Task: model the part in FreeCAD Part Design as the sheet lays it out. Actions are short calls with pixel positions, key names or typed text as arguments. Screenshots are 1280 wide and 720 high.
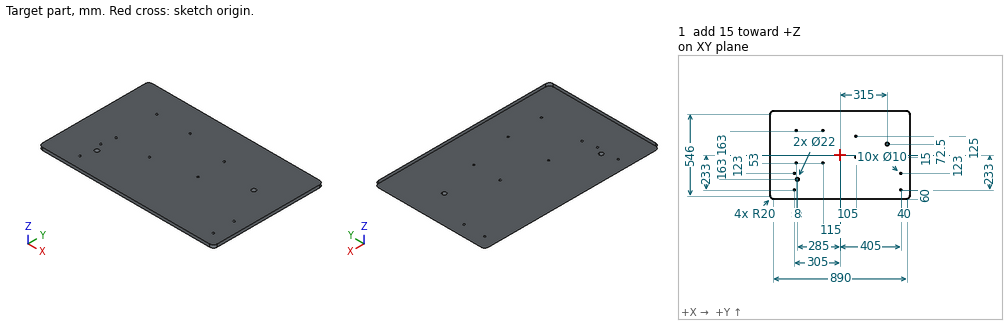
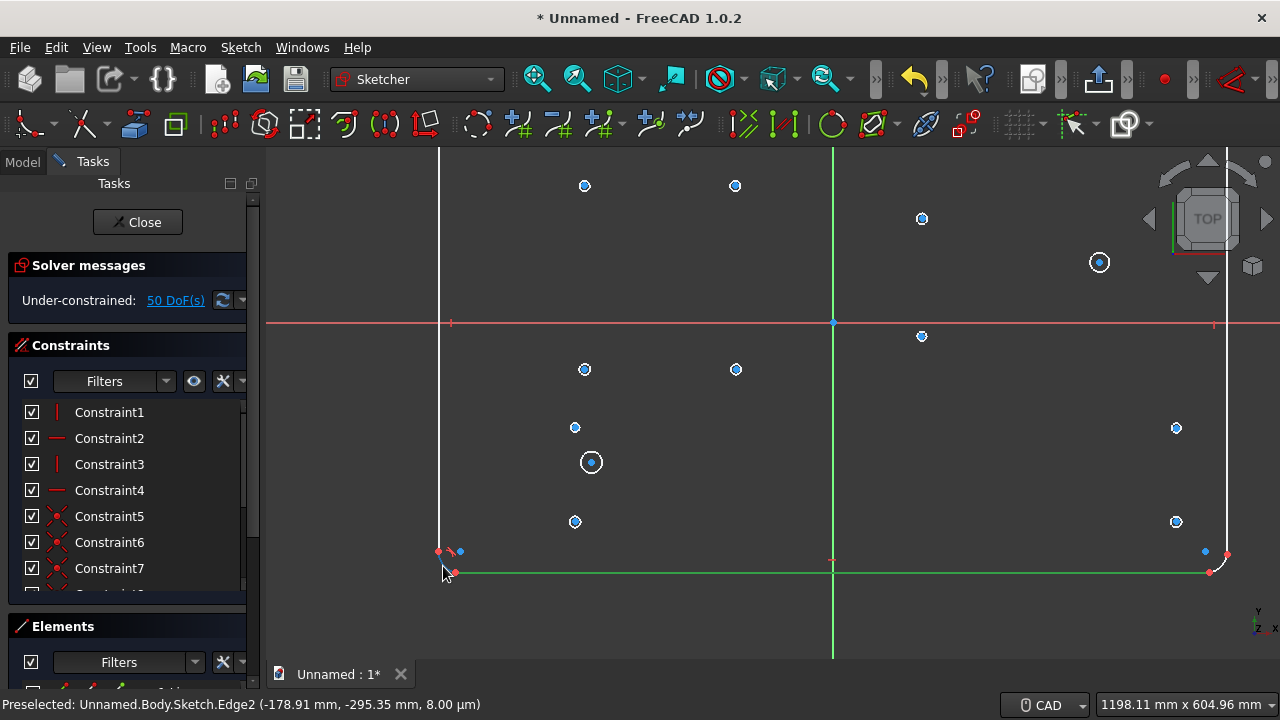
click(443, 565)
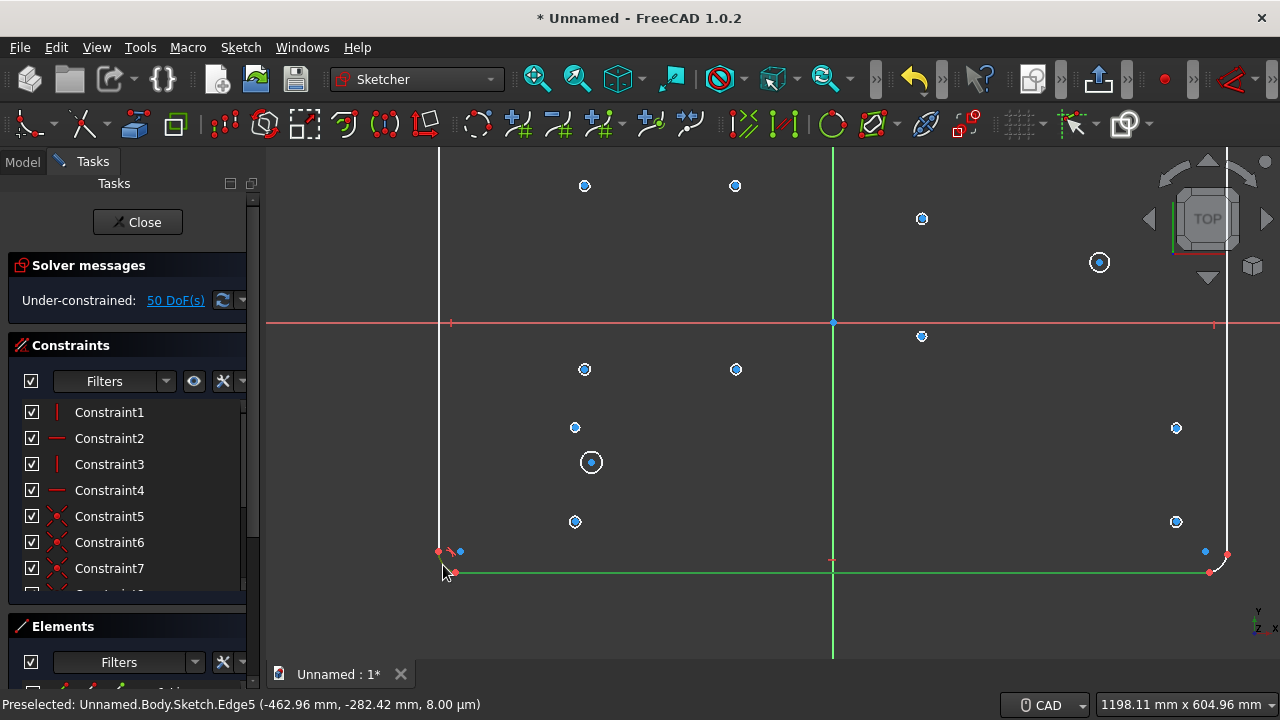
key(t)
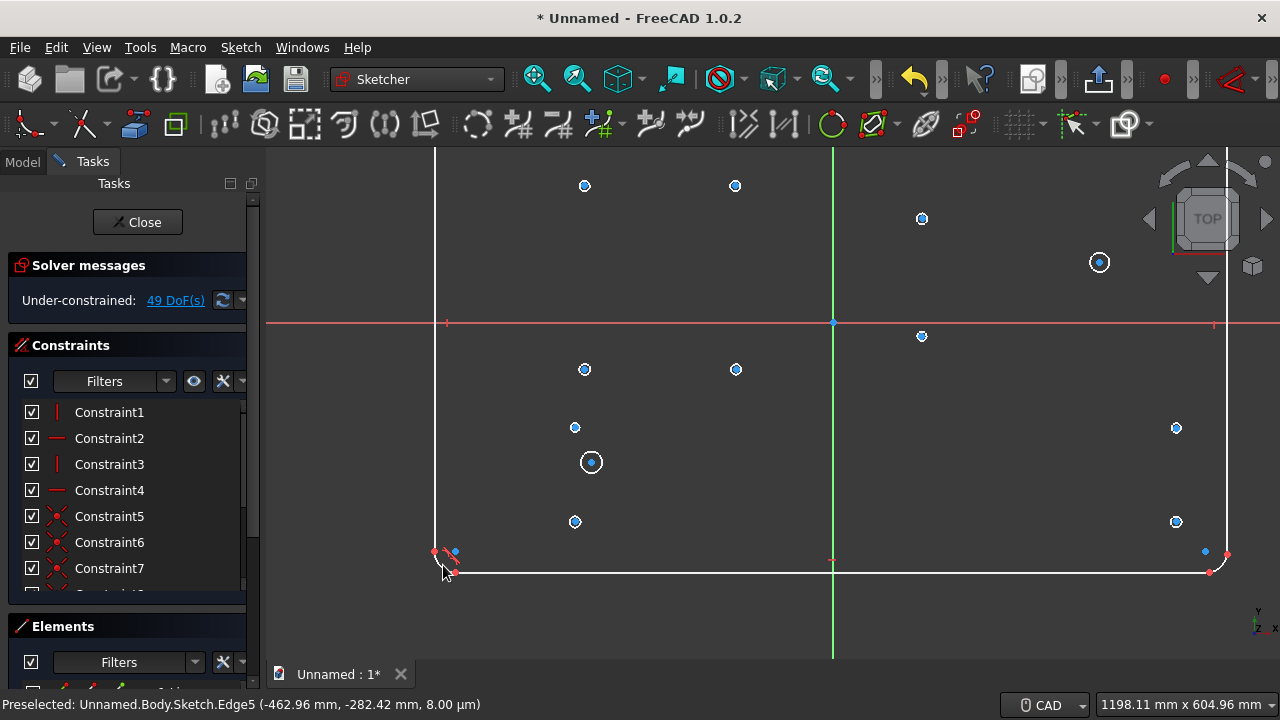
click(682, 573)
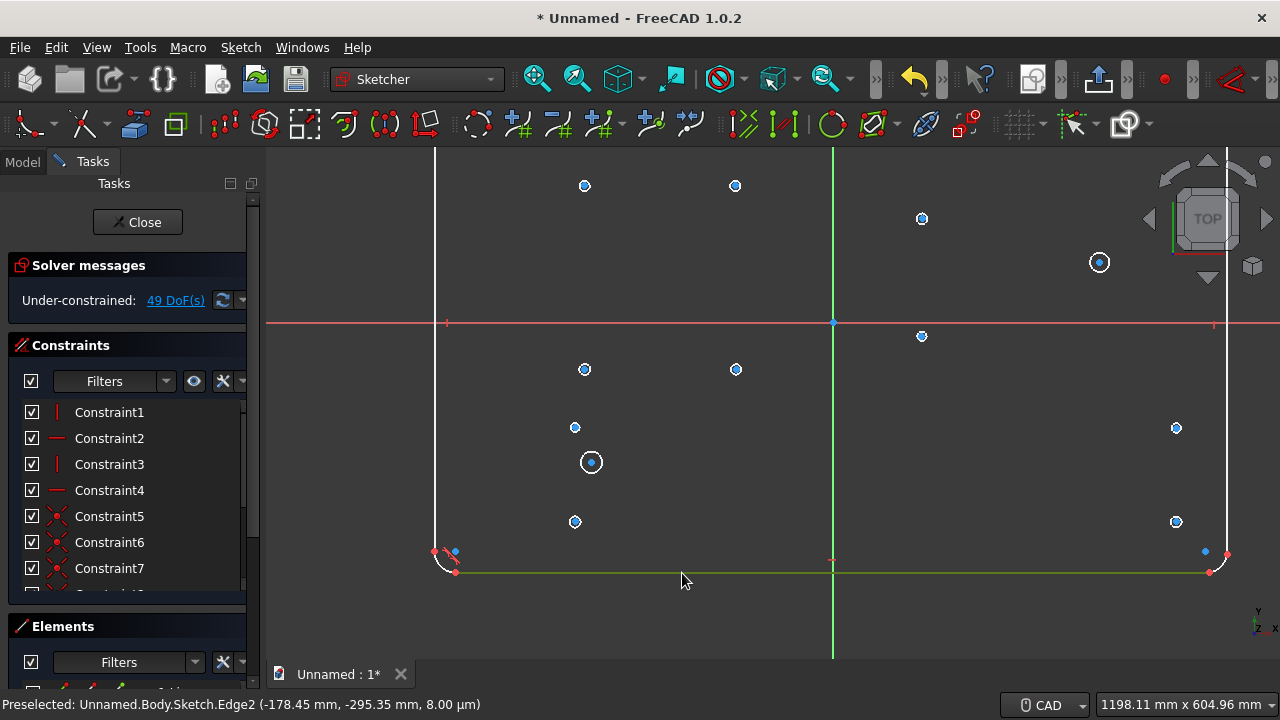
scroll(443, 566, down, 2)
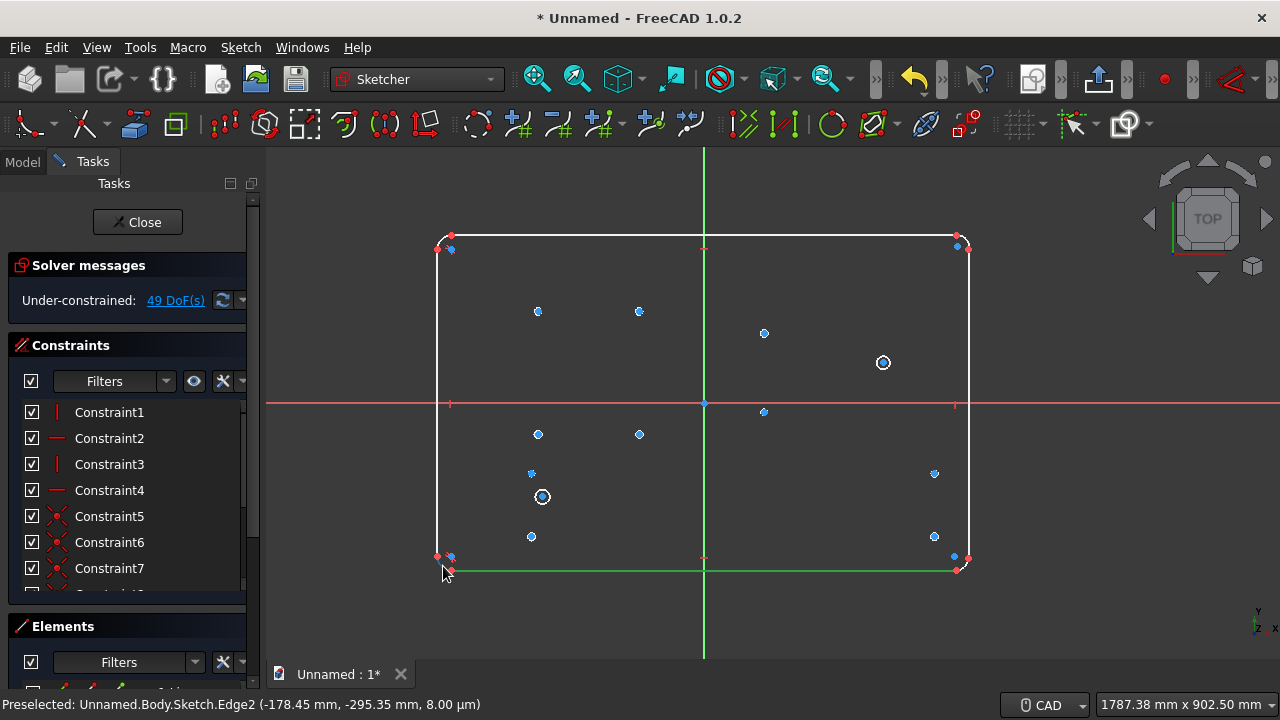
scroll(965, 567, up, 3)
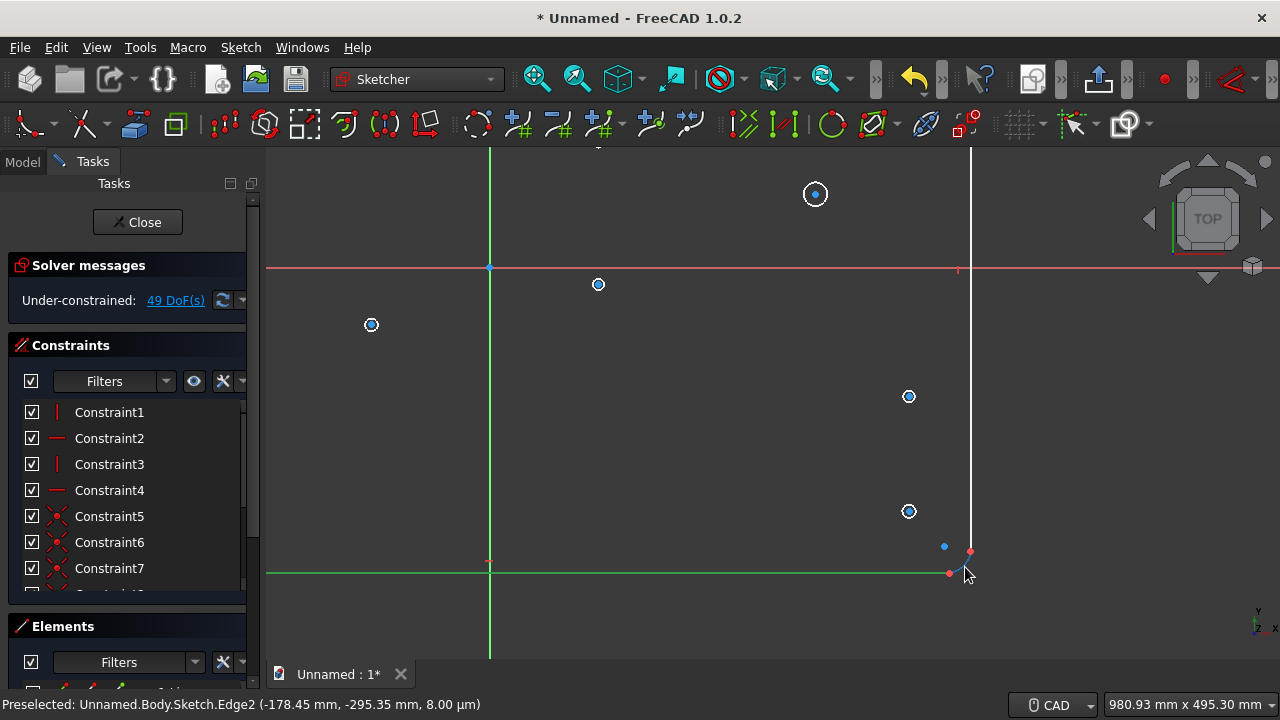
click(964, 566)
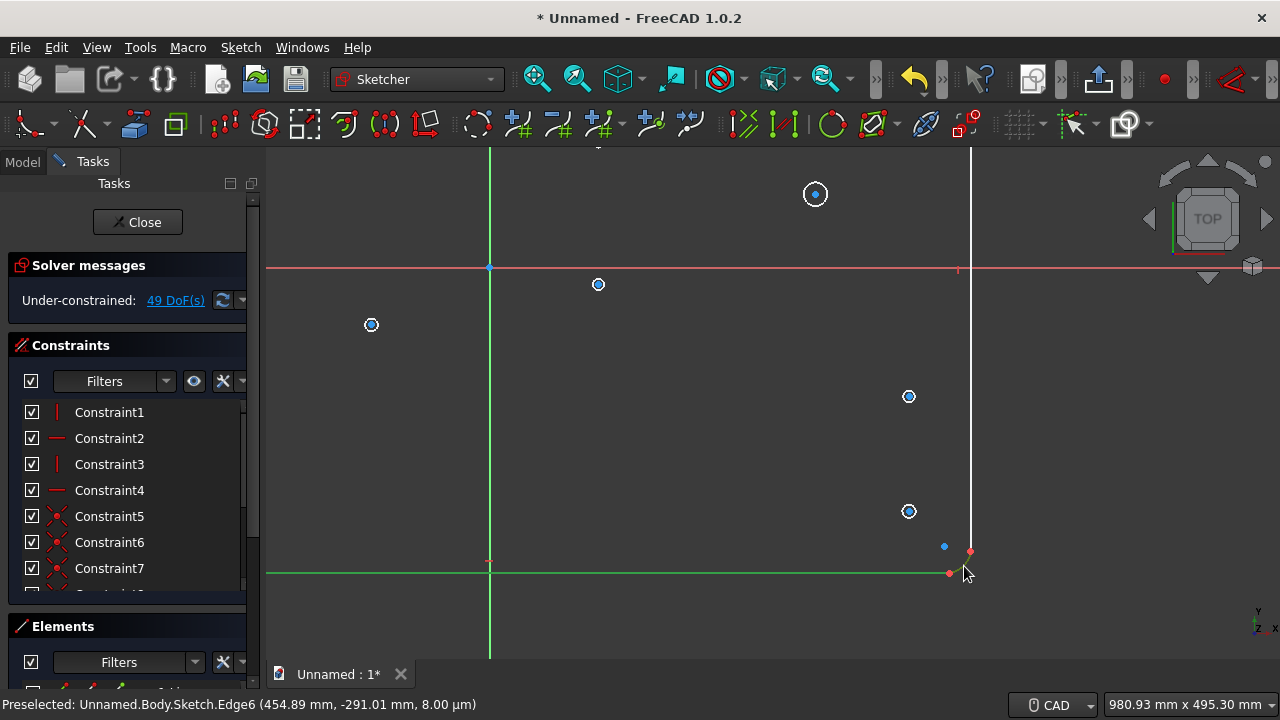
key(t)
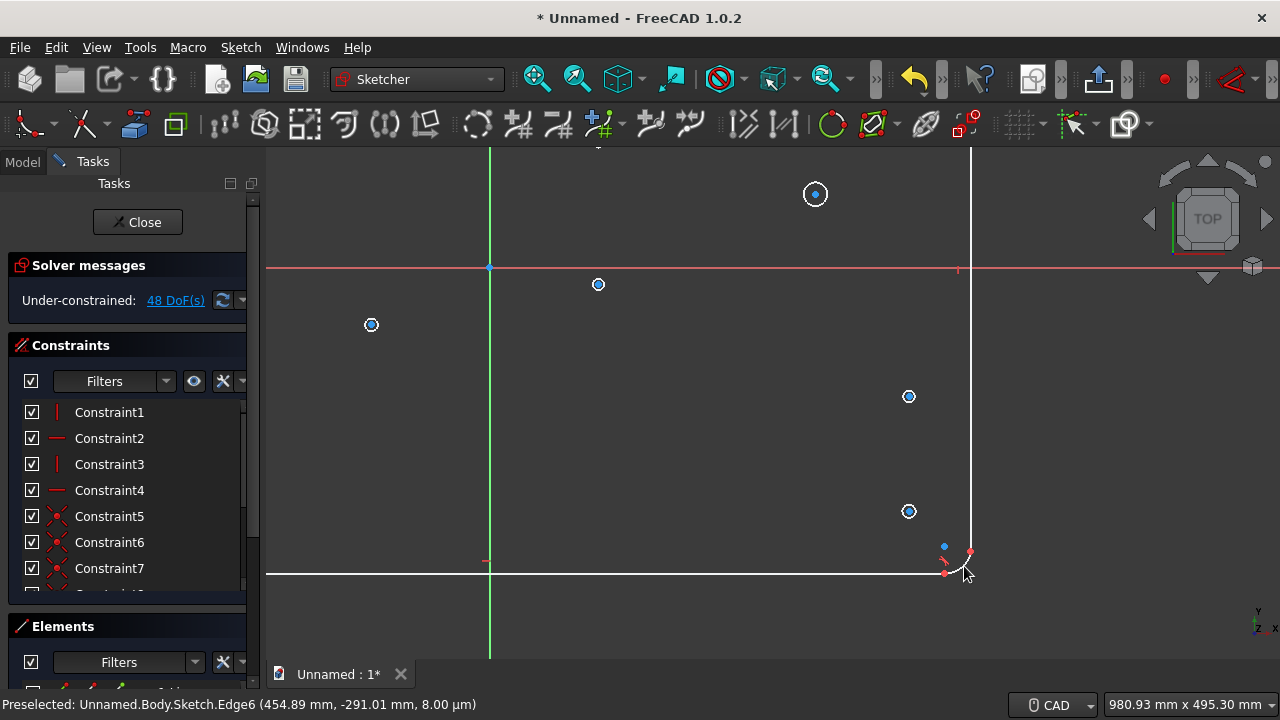
click(971, 382)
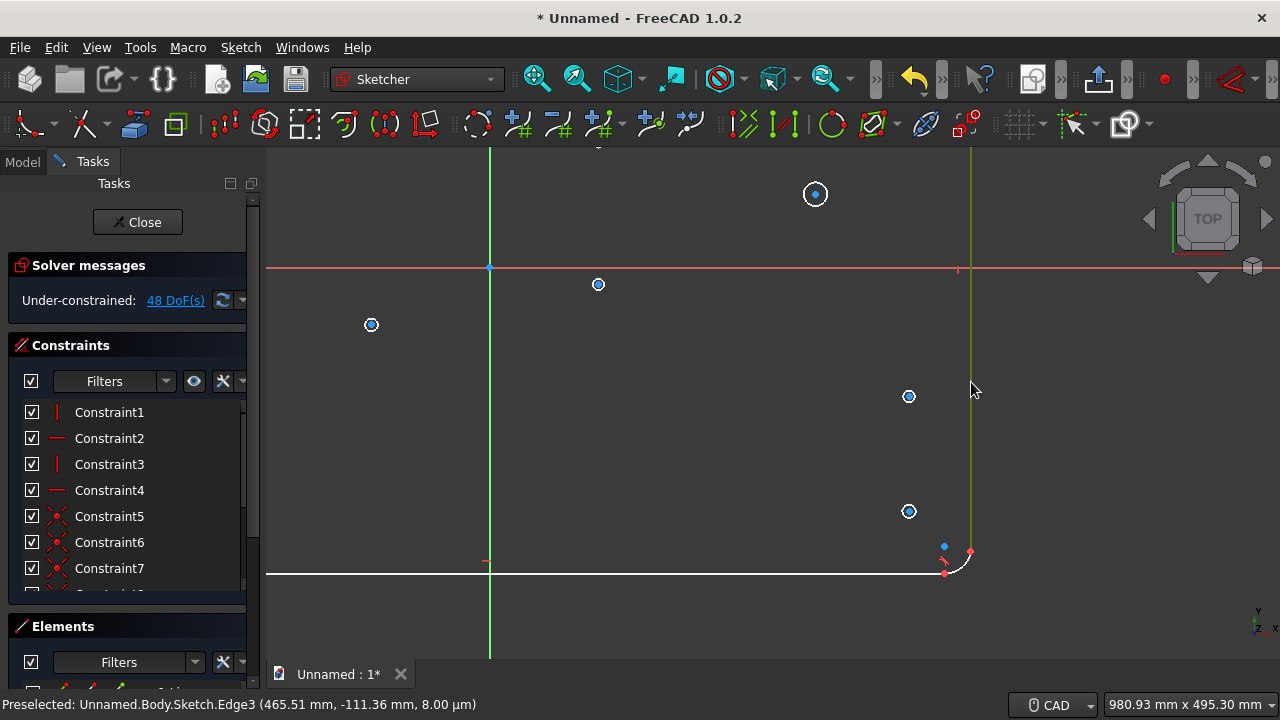
scroll(956, 571, up, 2)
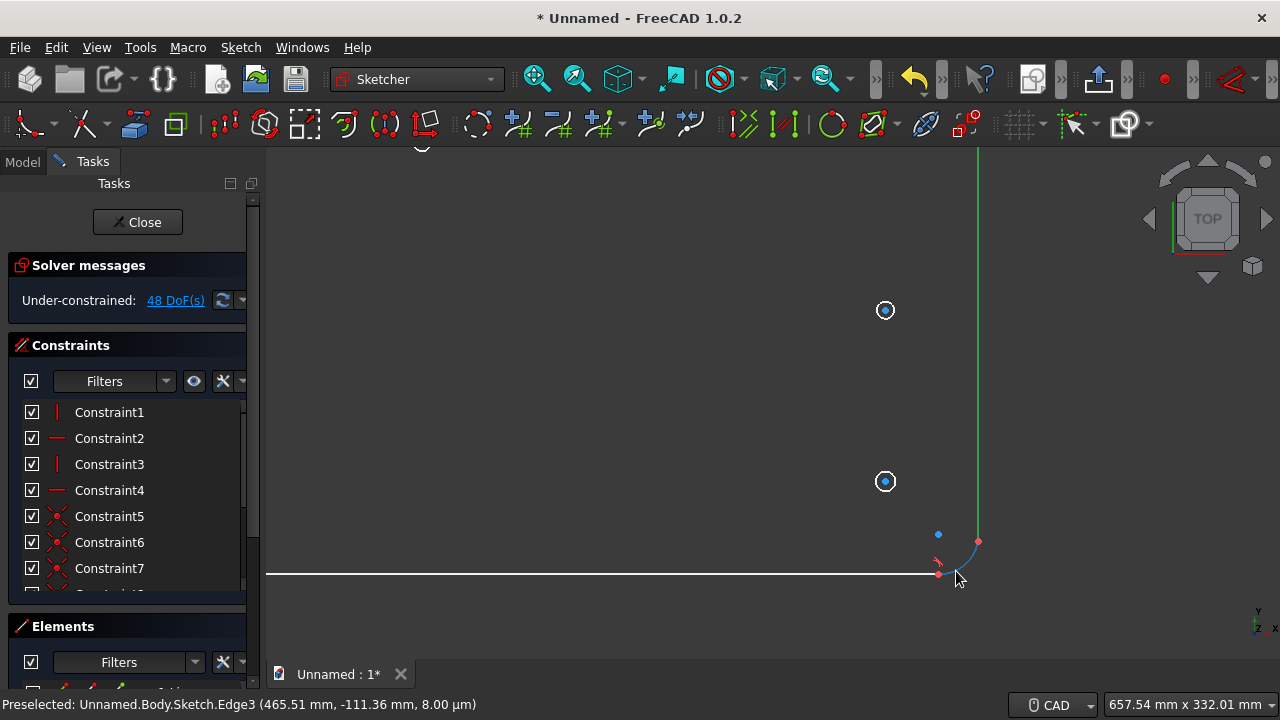
click(955, 571)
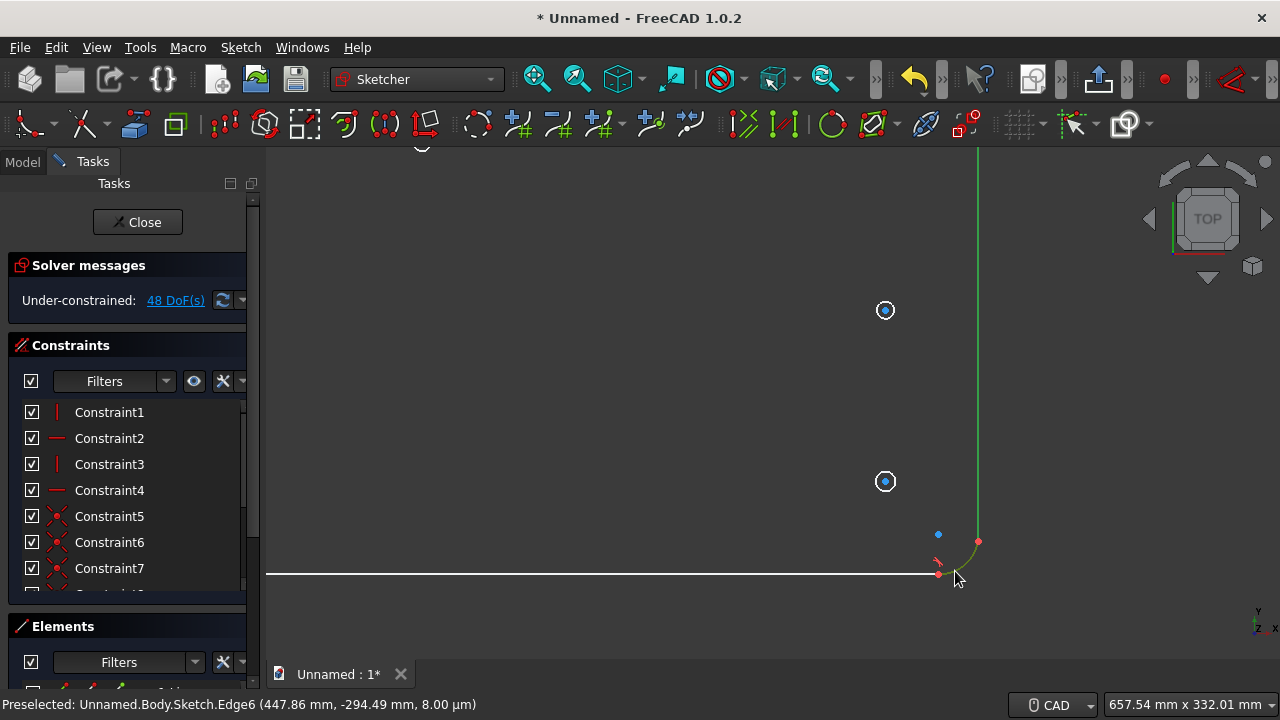
key(t)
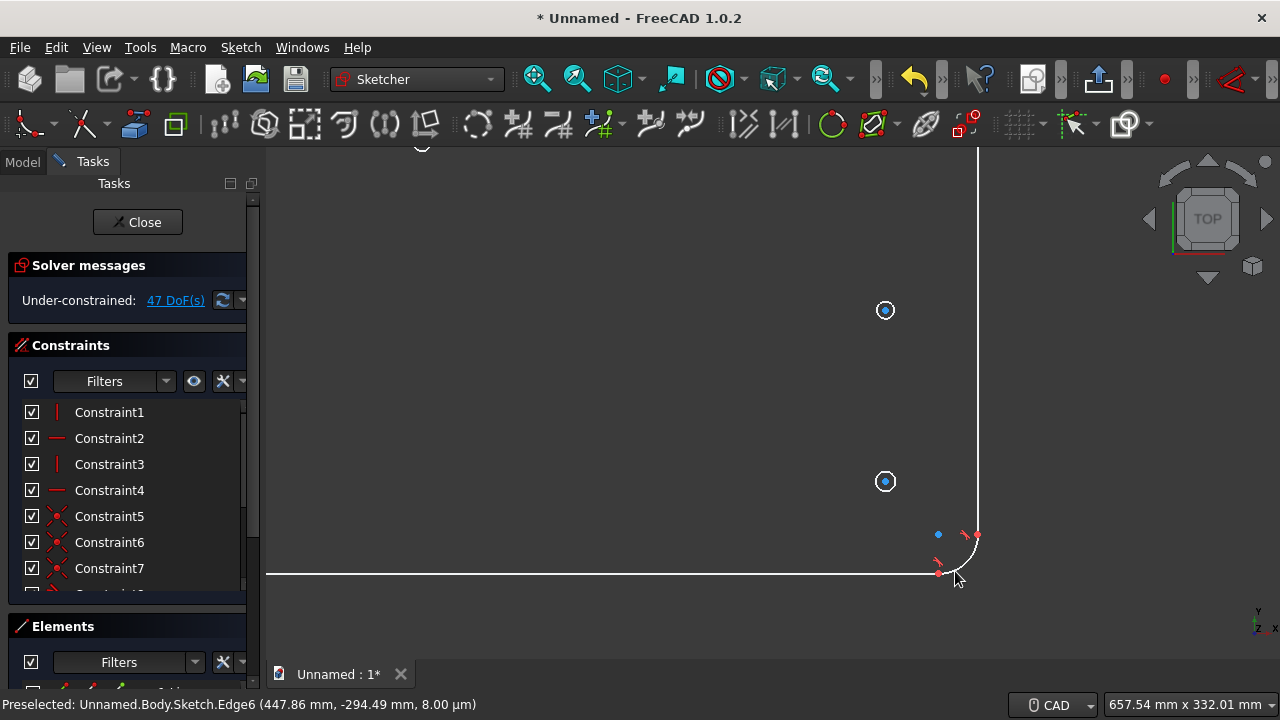
click(978, 285)